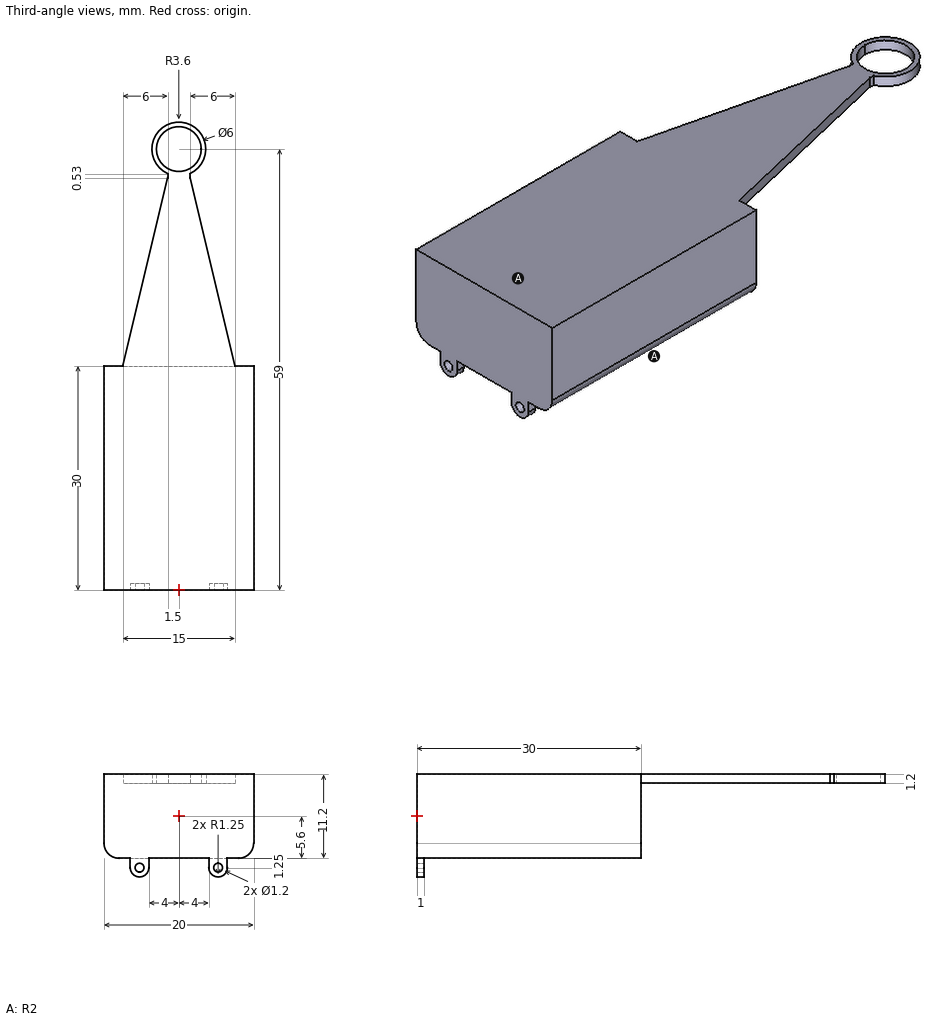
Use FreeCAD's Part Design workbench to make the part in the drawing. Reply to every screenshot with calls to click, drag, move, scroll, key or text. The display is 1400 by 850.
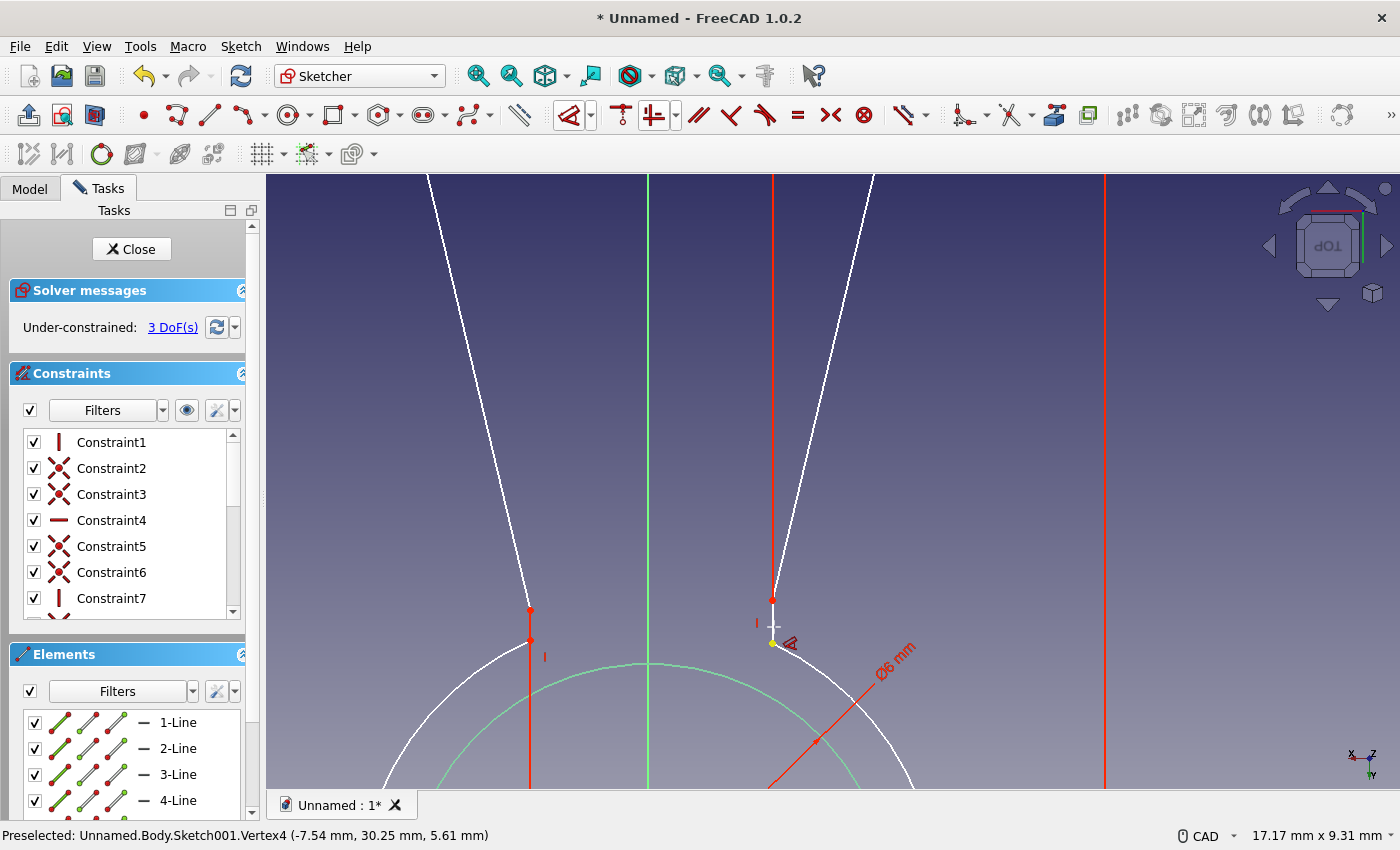
click(773, 622)
click(807, 622)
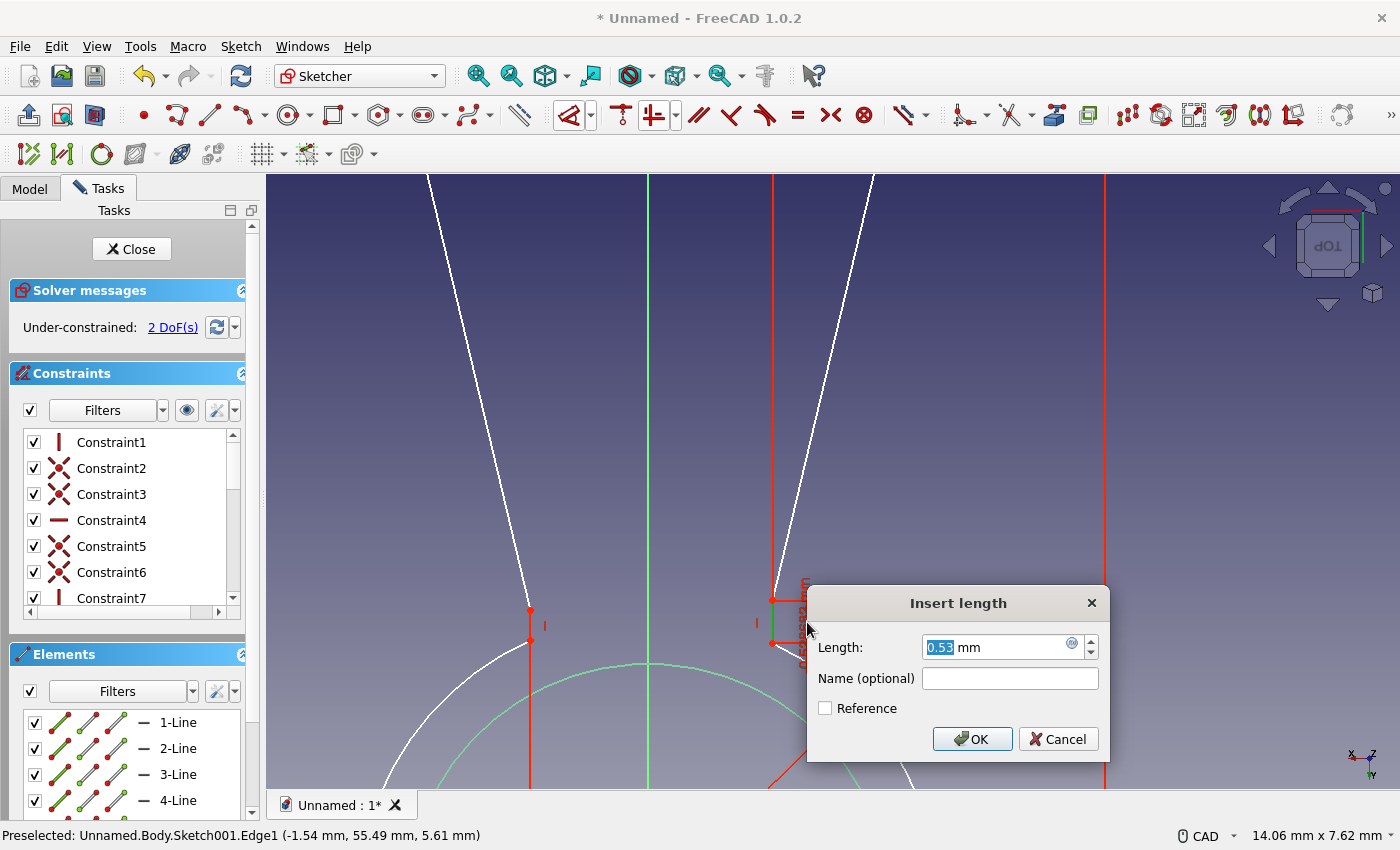
text(0.53)
key(Return)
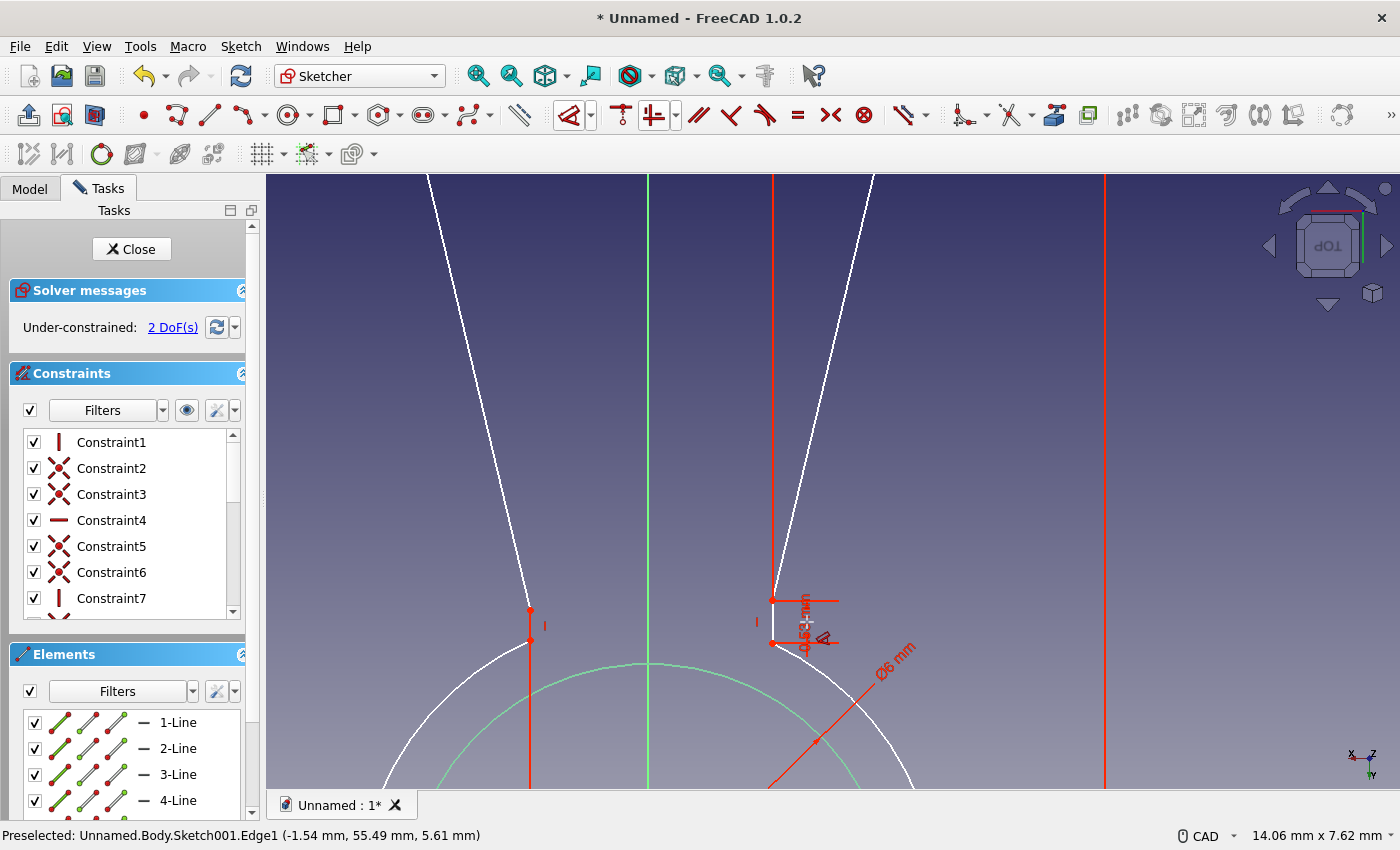
click(530, 619)
click(496, 625)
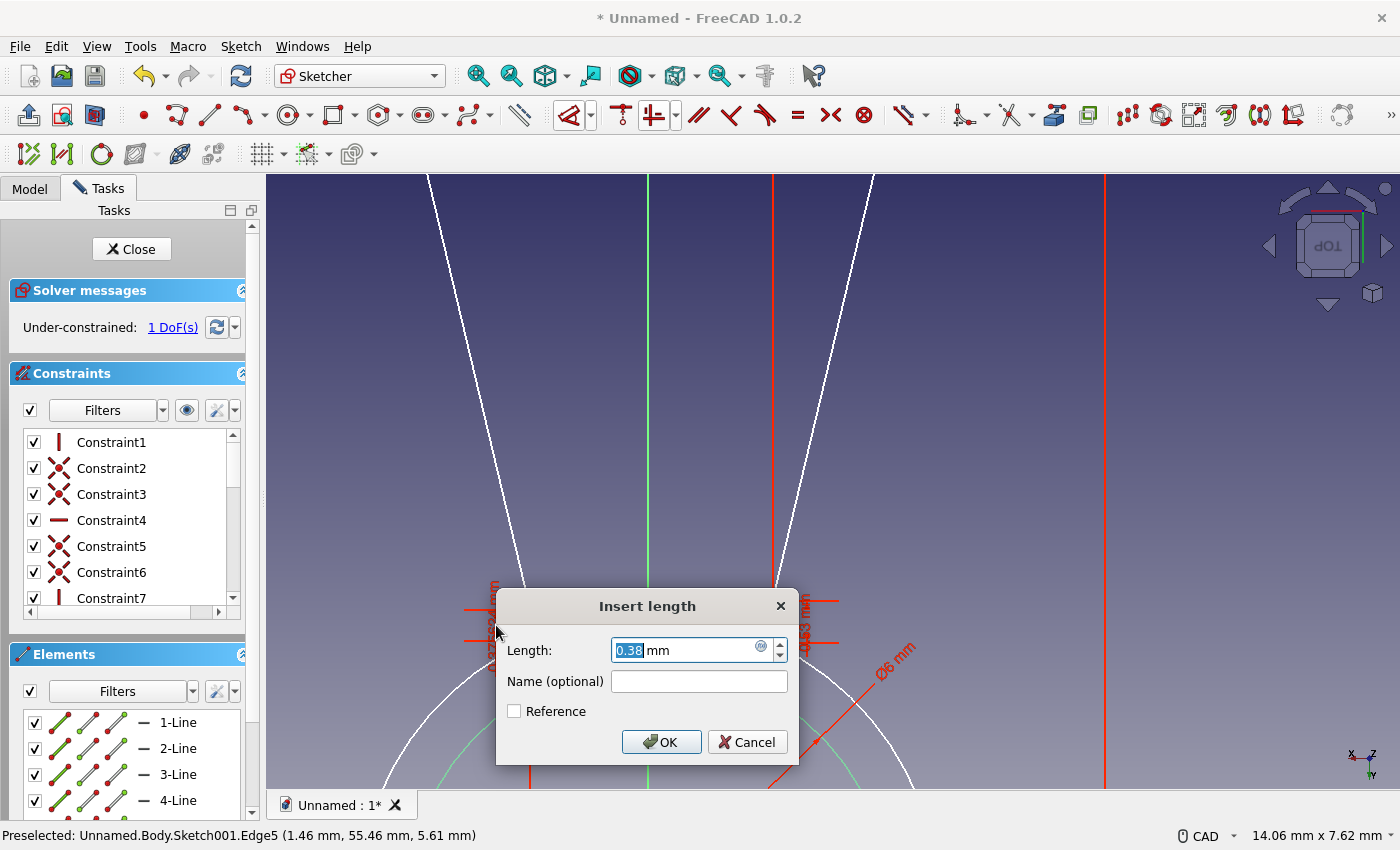
text(0.53)
key(Return)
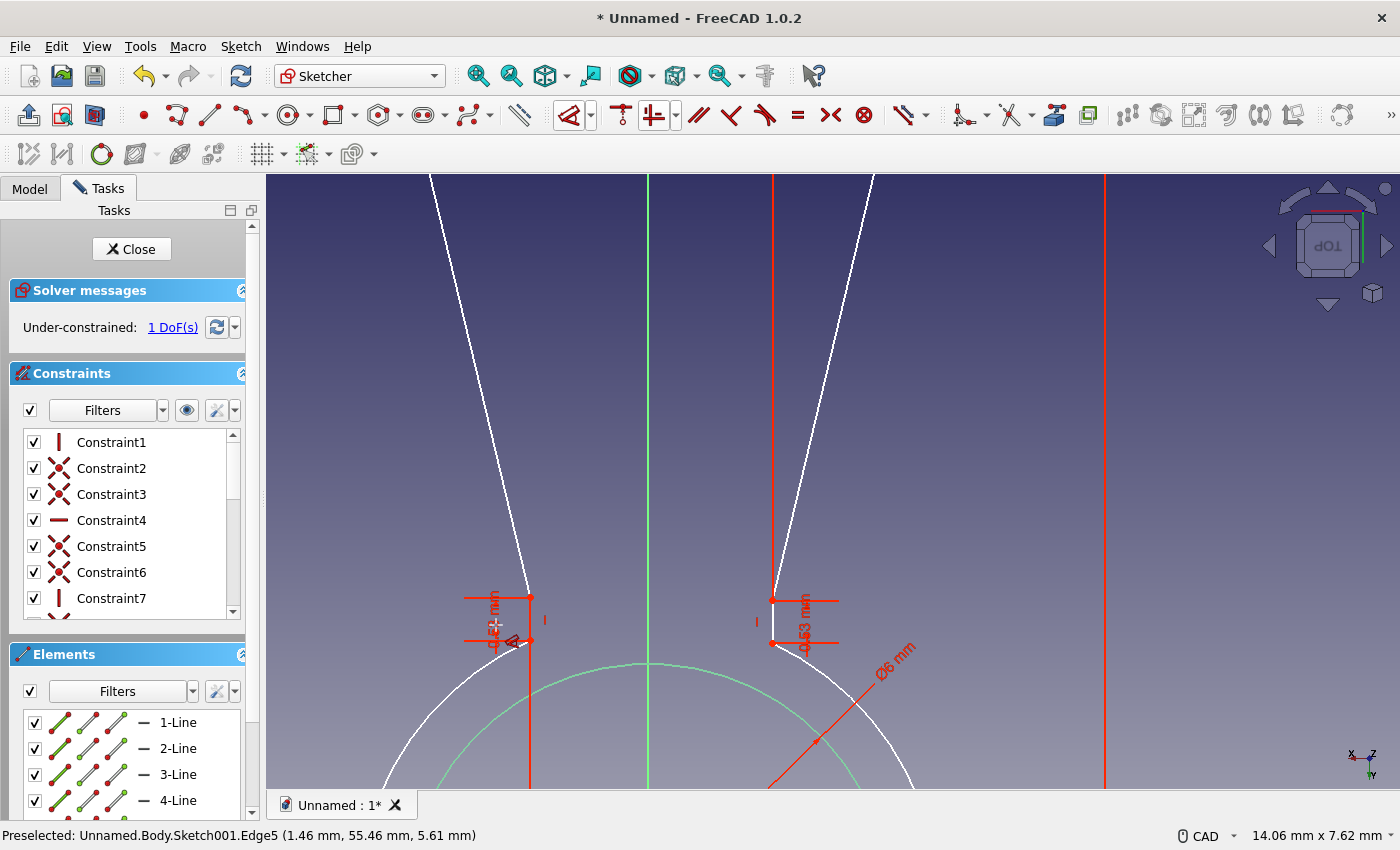
scroll(774, 627, down, 13)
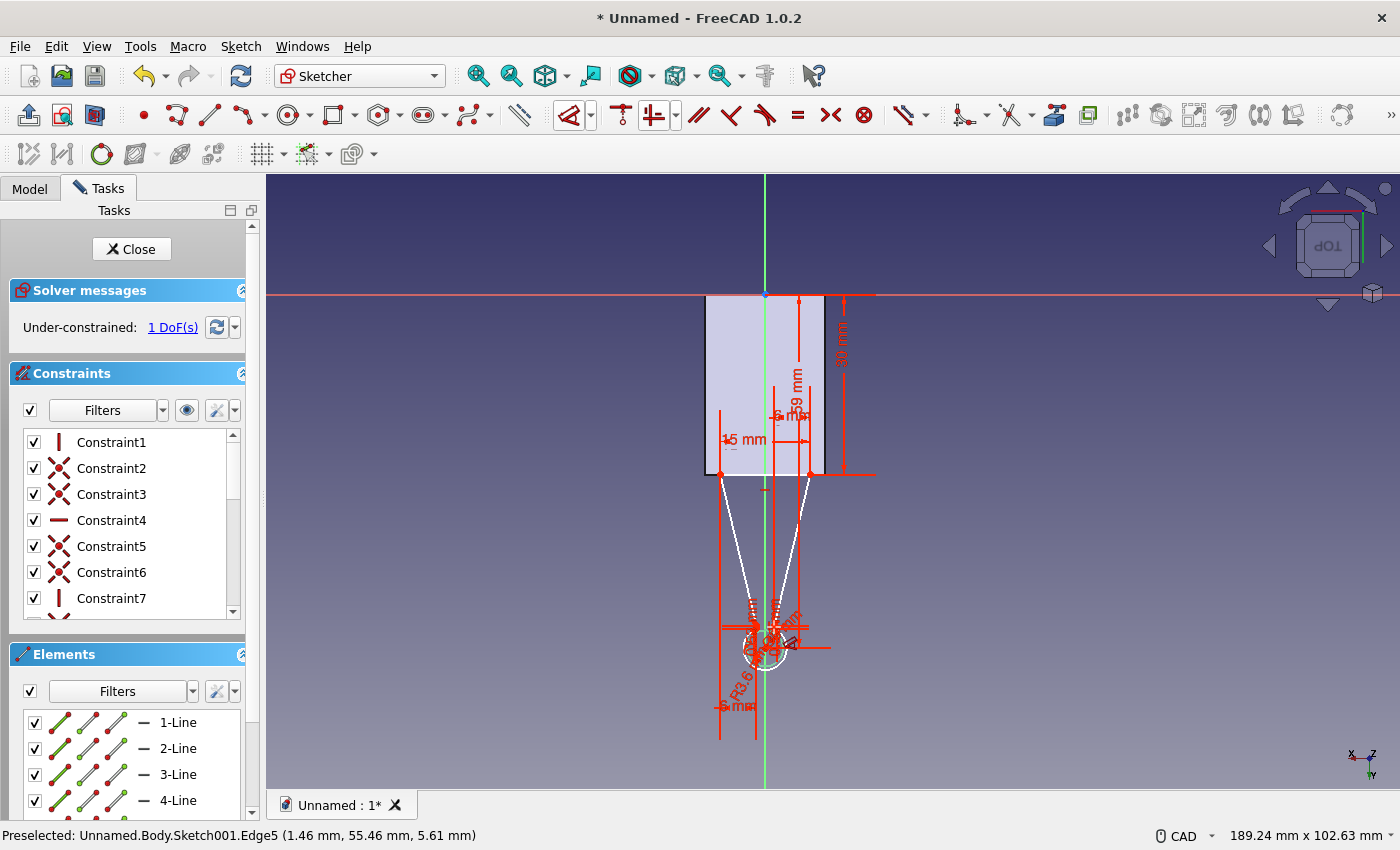
scroll(774, 629, up, 8)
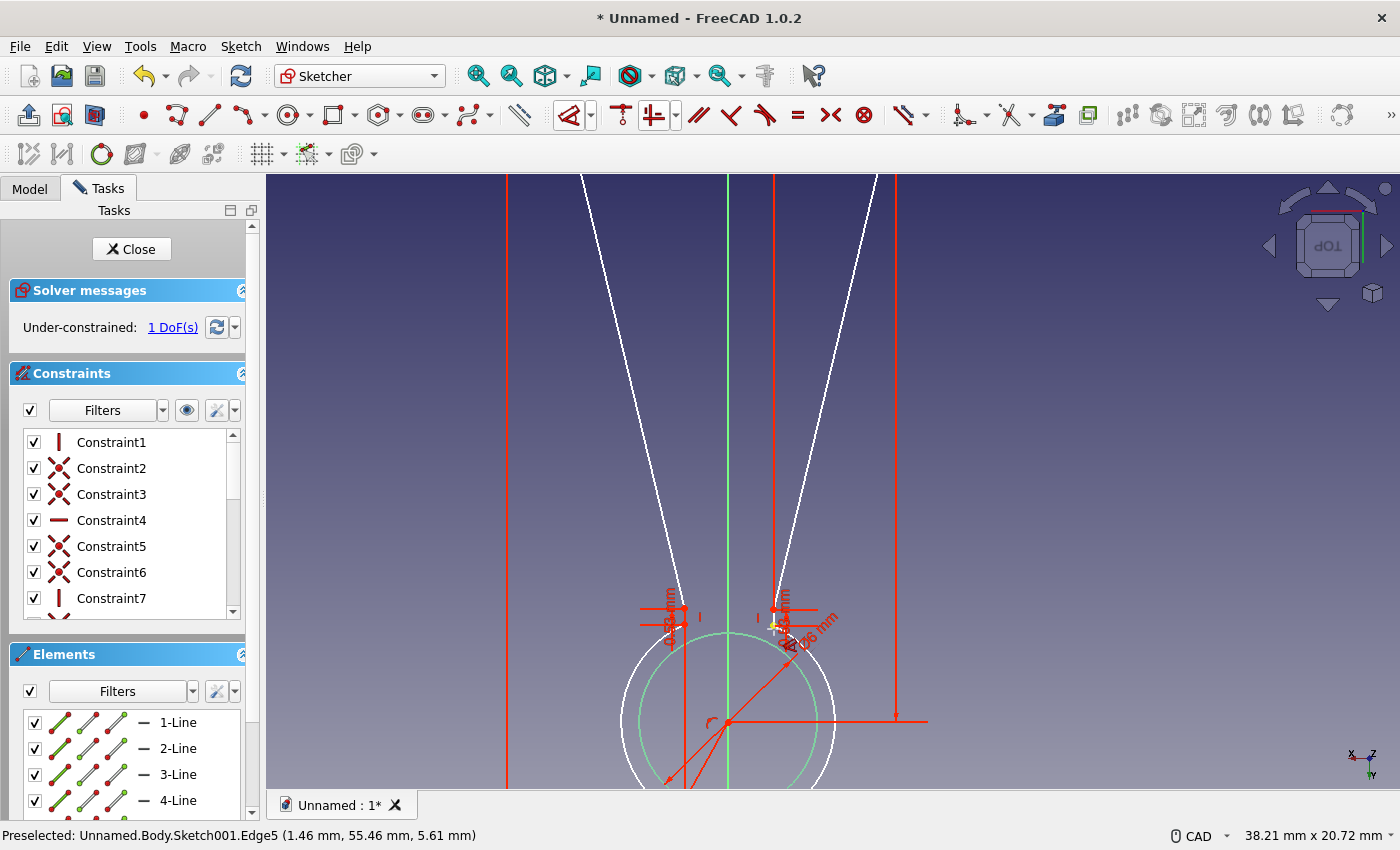
click(774, 626)
click(751, 660)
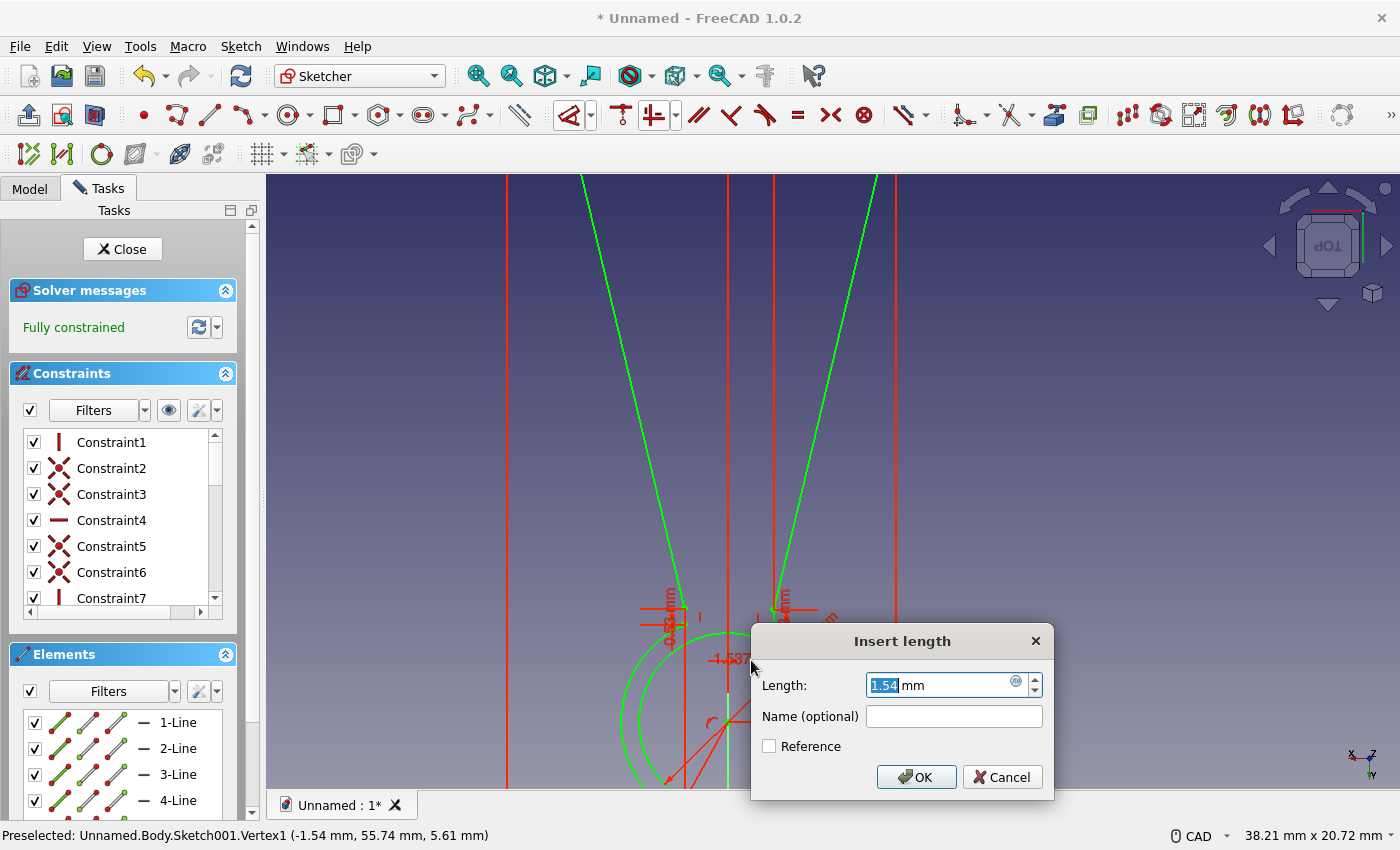
text(1.5)
key(Return)
key(Escape)